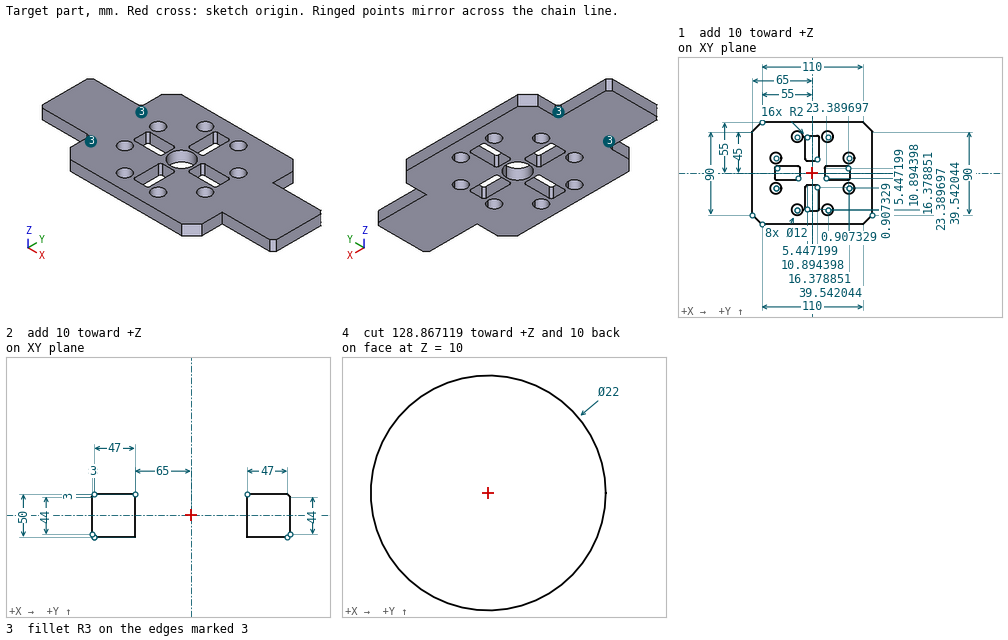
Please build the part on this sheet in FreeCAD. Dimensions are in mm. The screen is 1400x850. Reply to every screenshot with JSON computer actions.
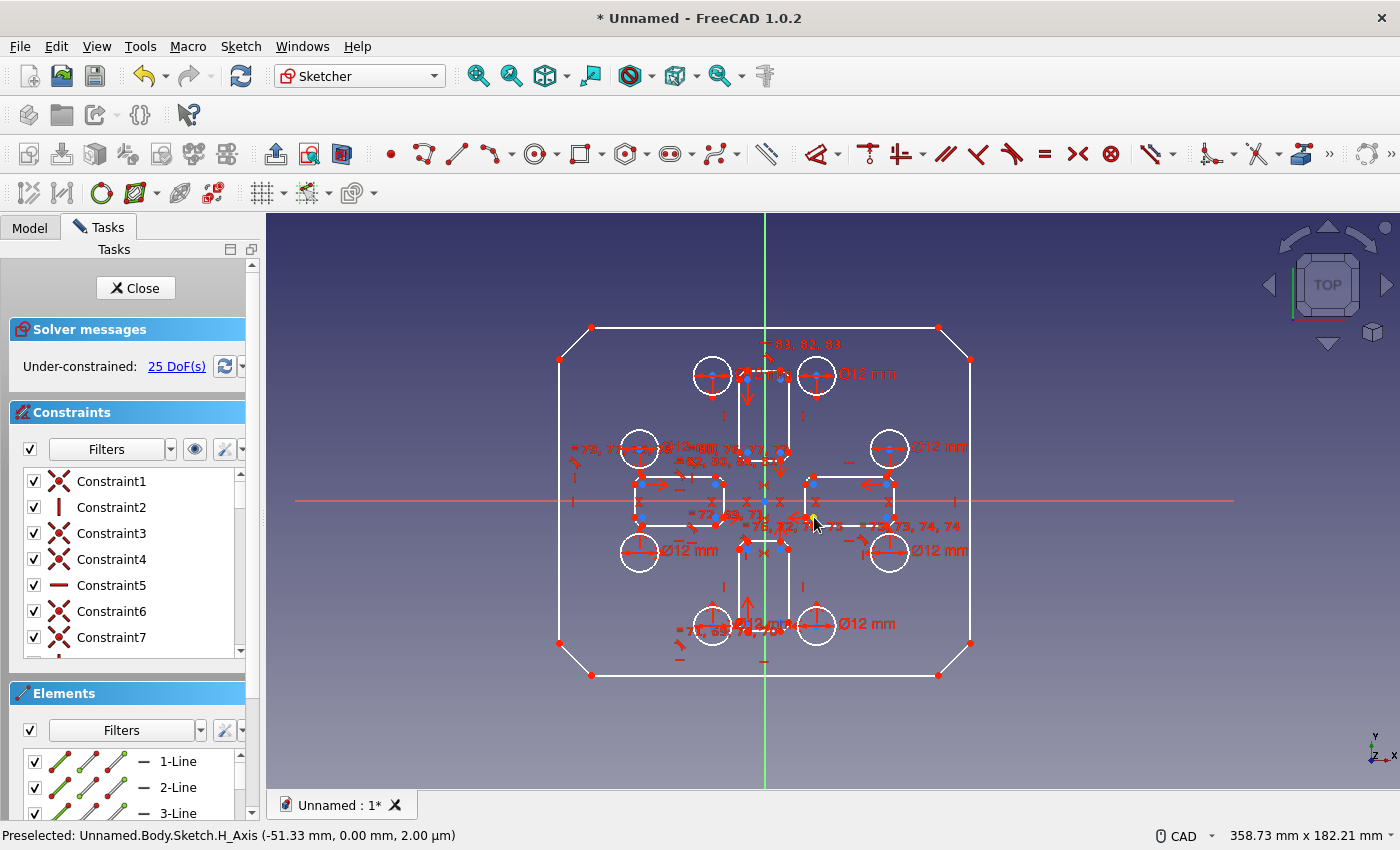
{"action": "left_click", "coordinate": [591, 328]}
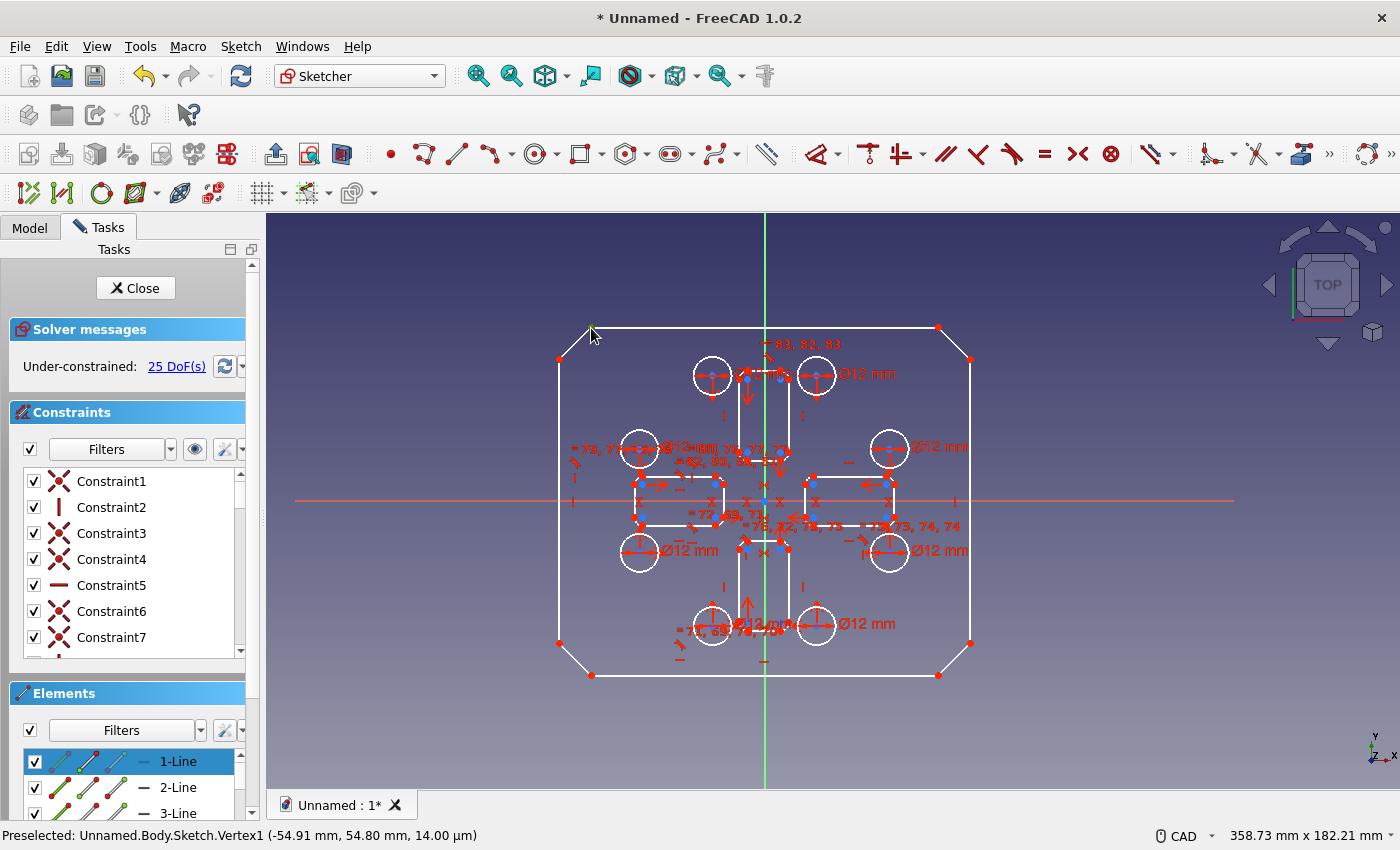
{"action": "left_click", "coordinate": [591, 676]}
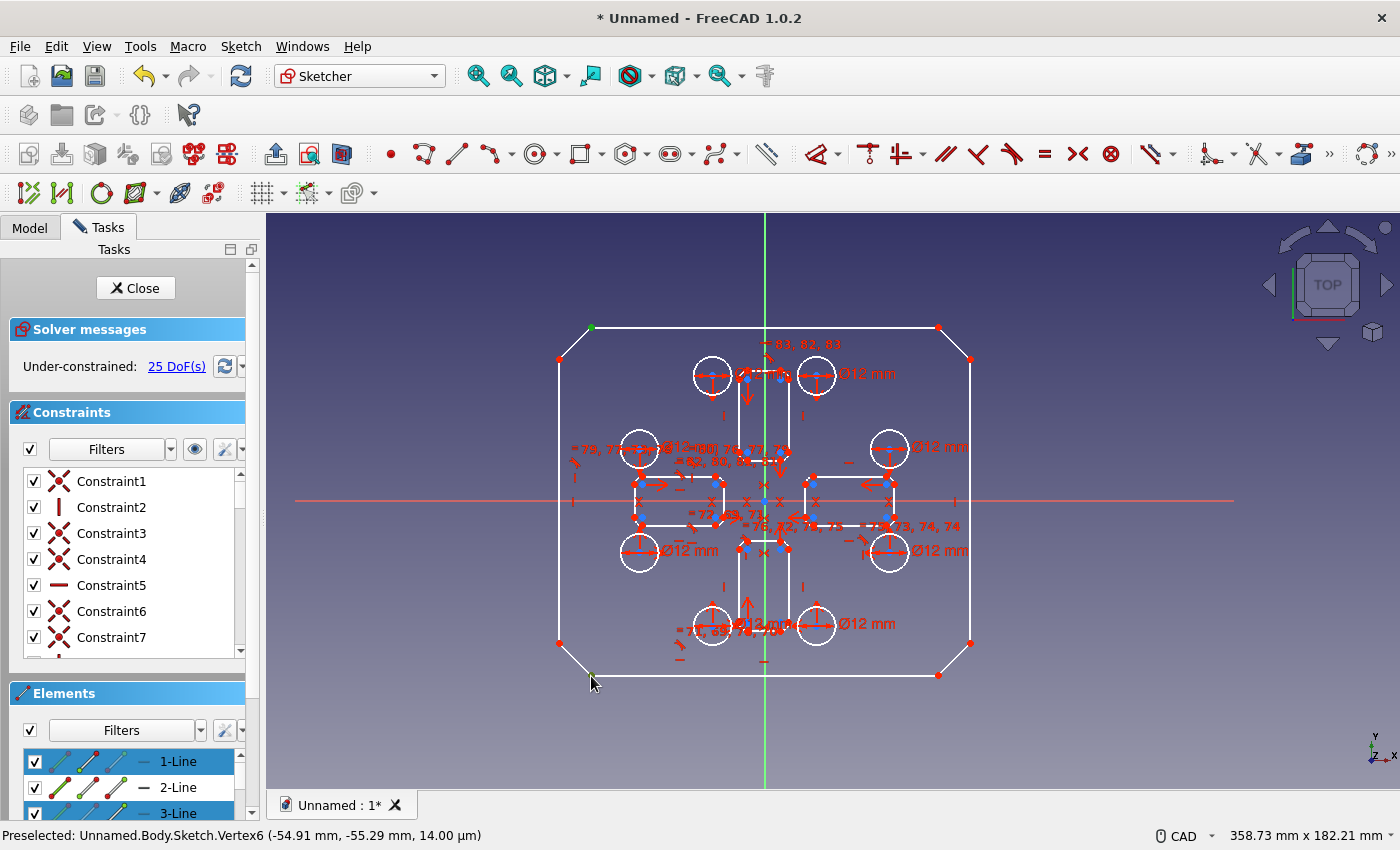
{"action": "left_click", "coordinate": [361, 501]}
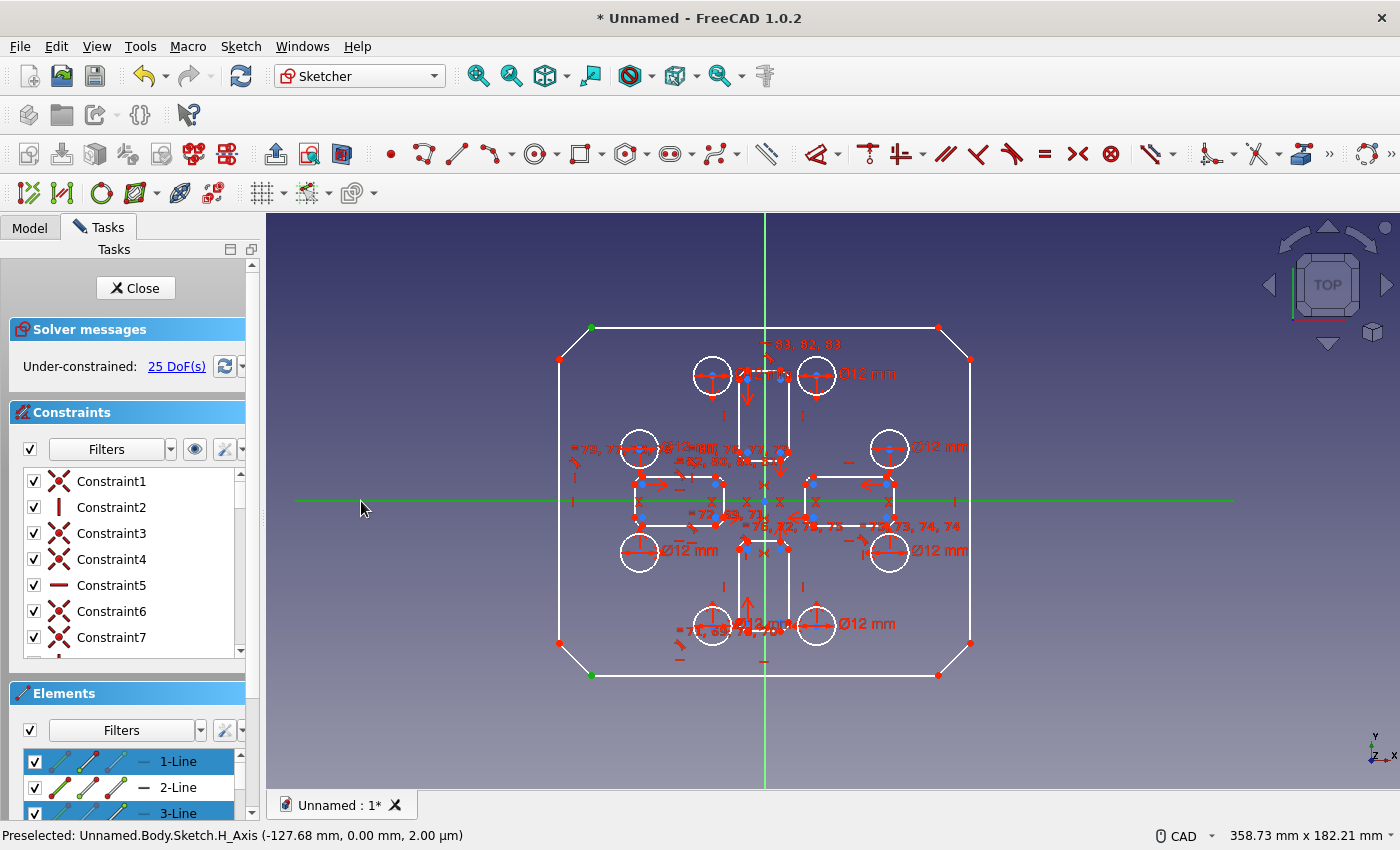
{"action": "left_click", "coordinate": [1078, 154]}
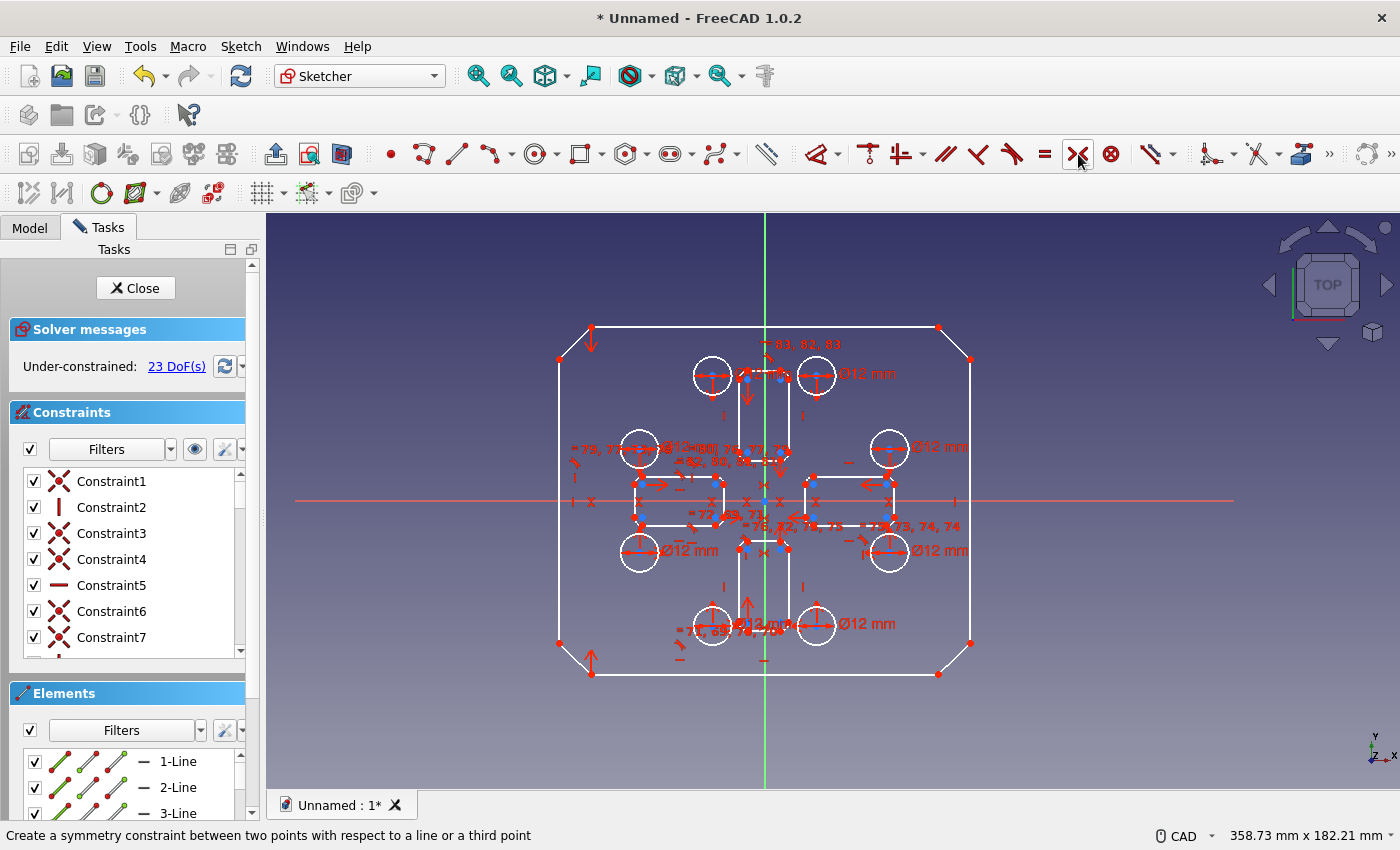
{"action": "left_click", "coordinate": [559, 644]}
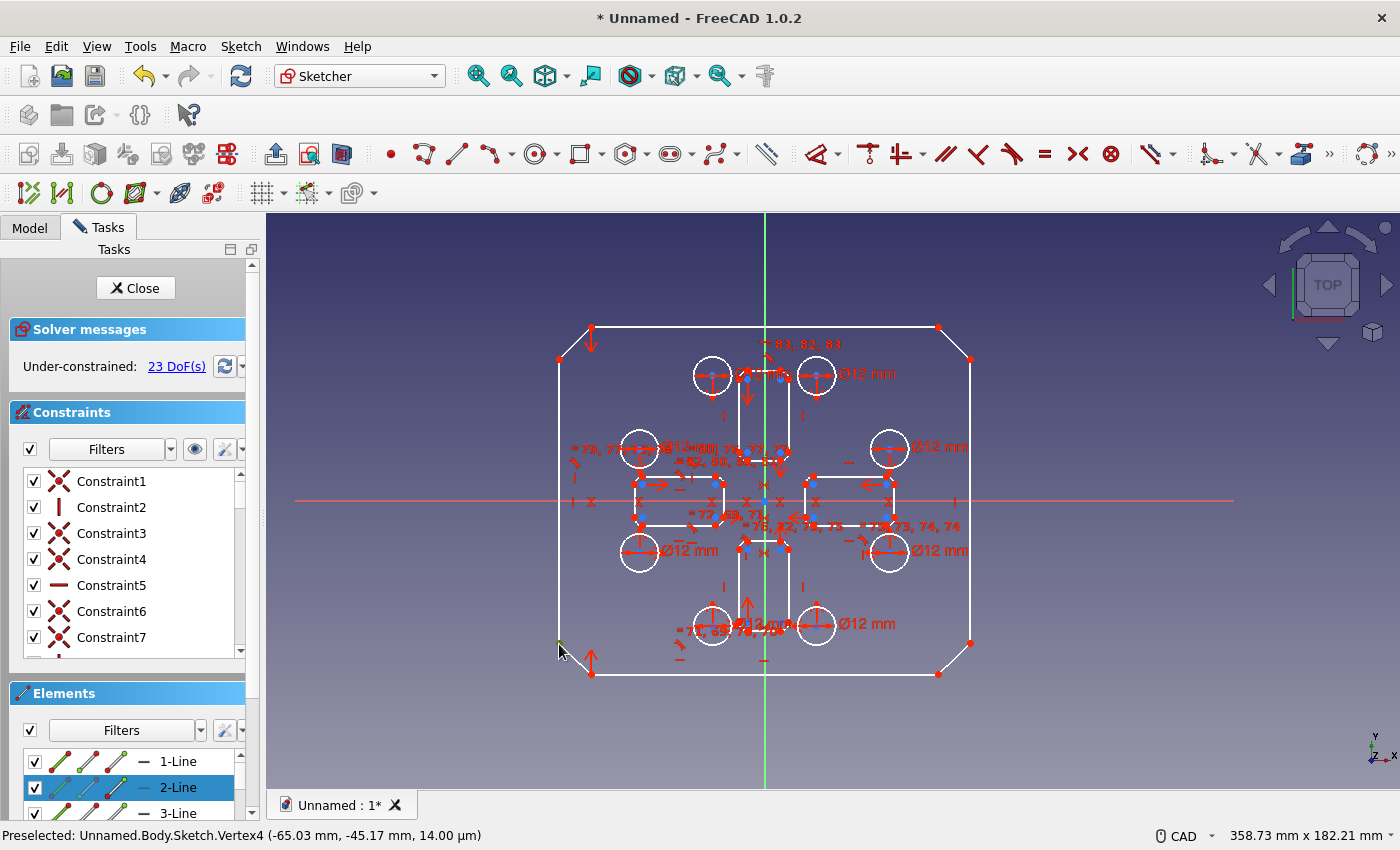
{"action": "left_click", "coordinate": [970, 644]}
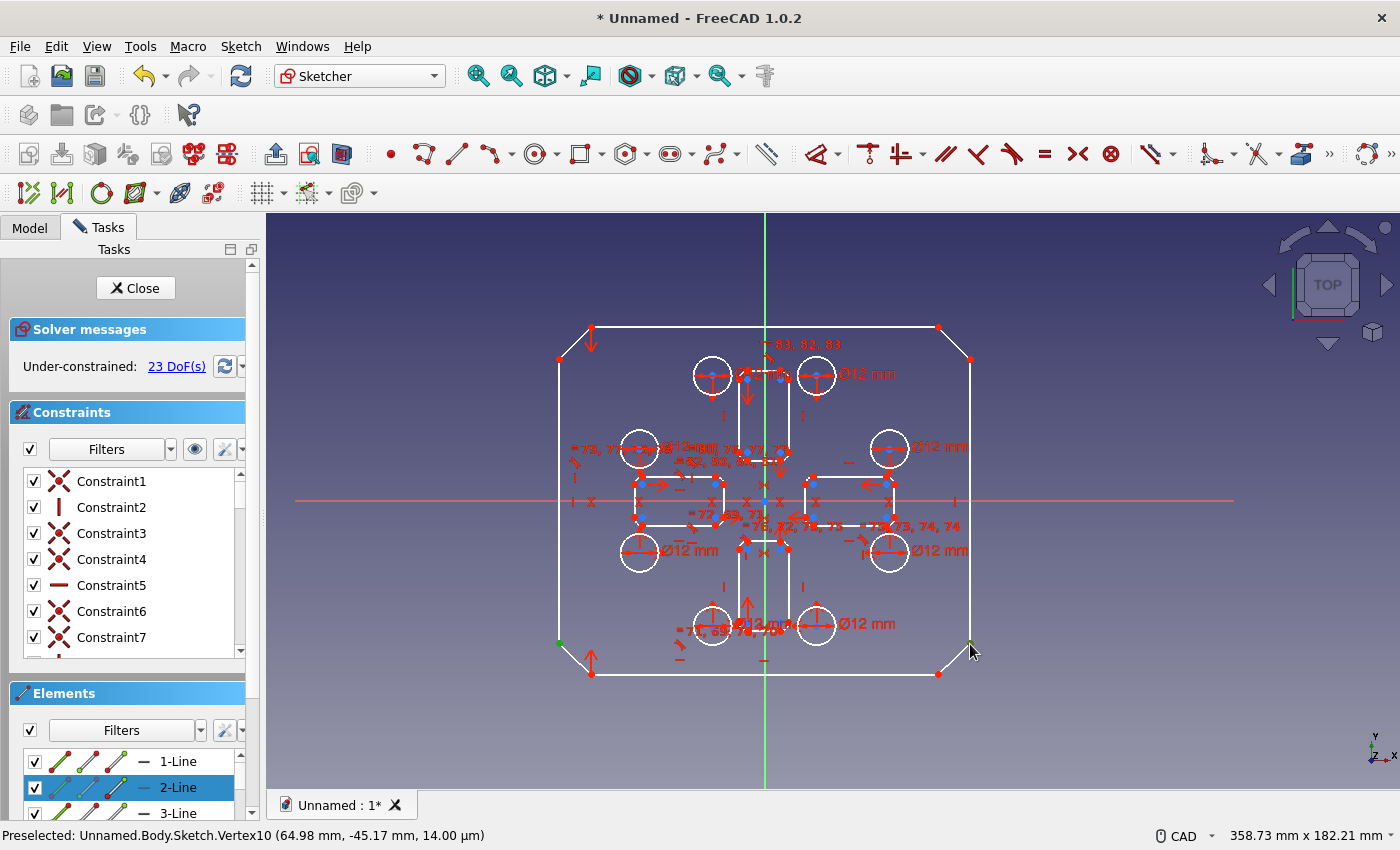
{"action": "left_click", "coordinate": [765, 724]}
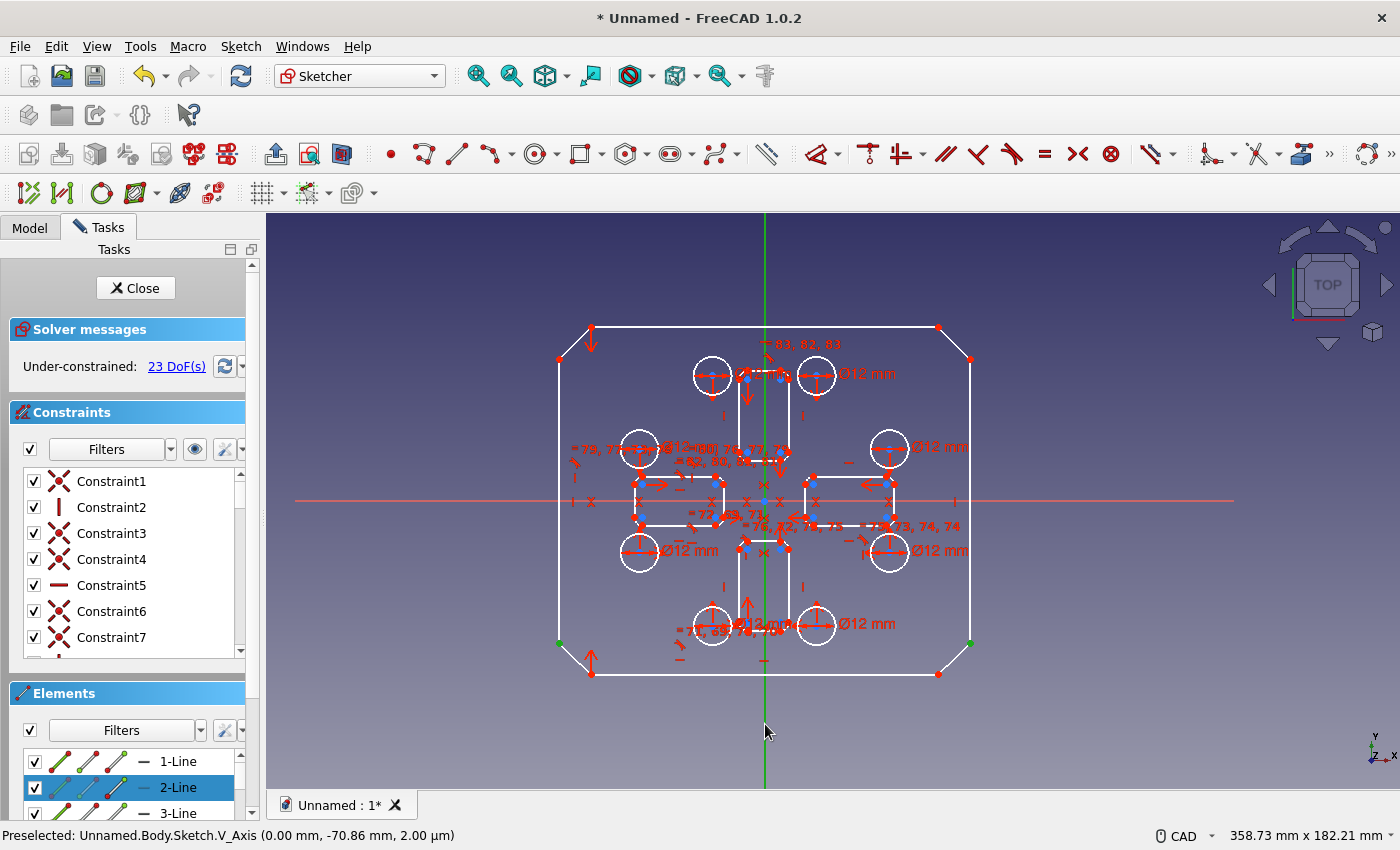
{"action": "left_click", "coordinate": [1078, 154]}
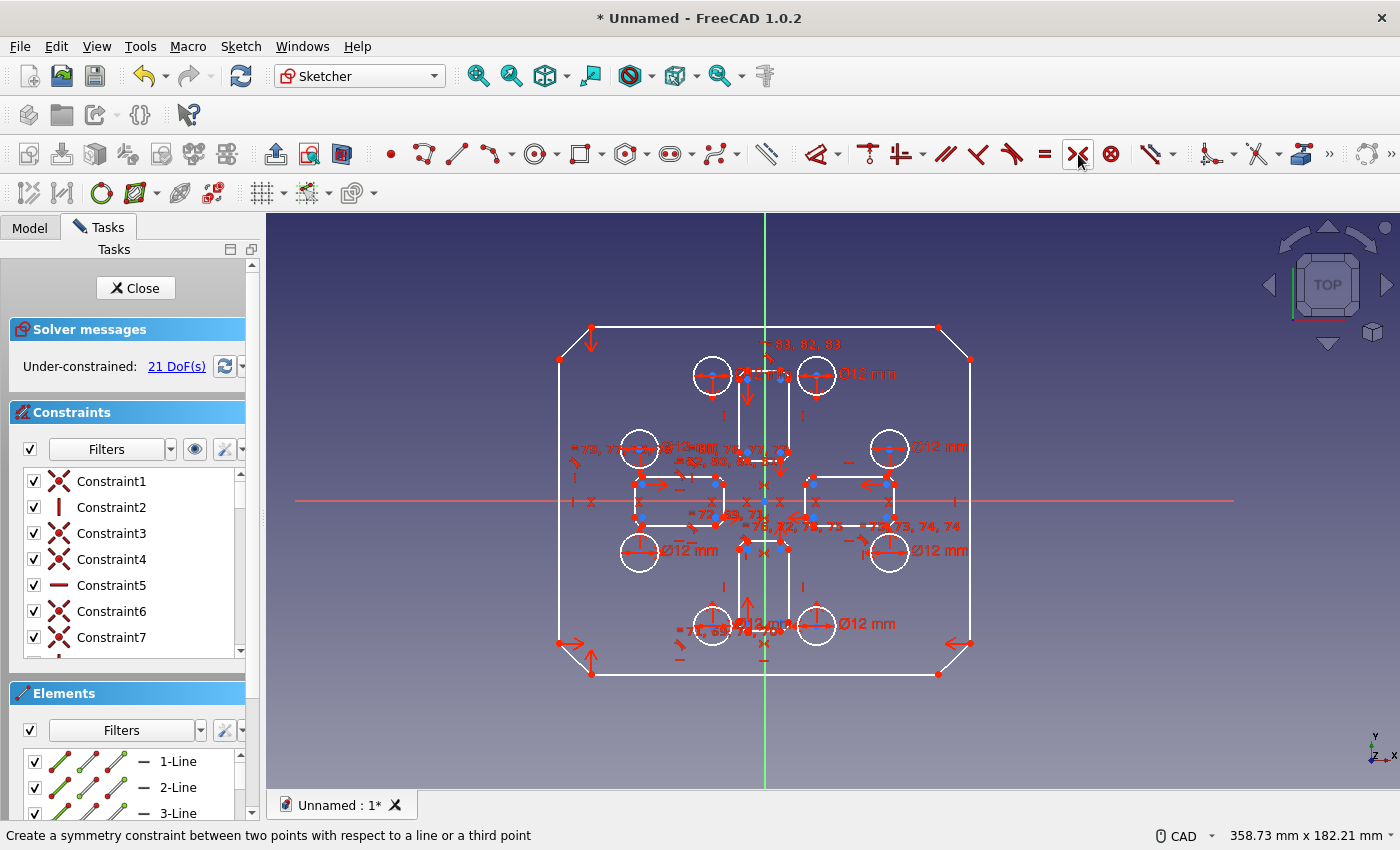
{"action": "left_click", "coordinate": [816, 154]}